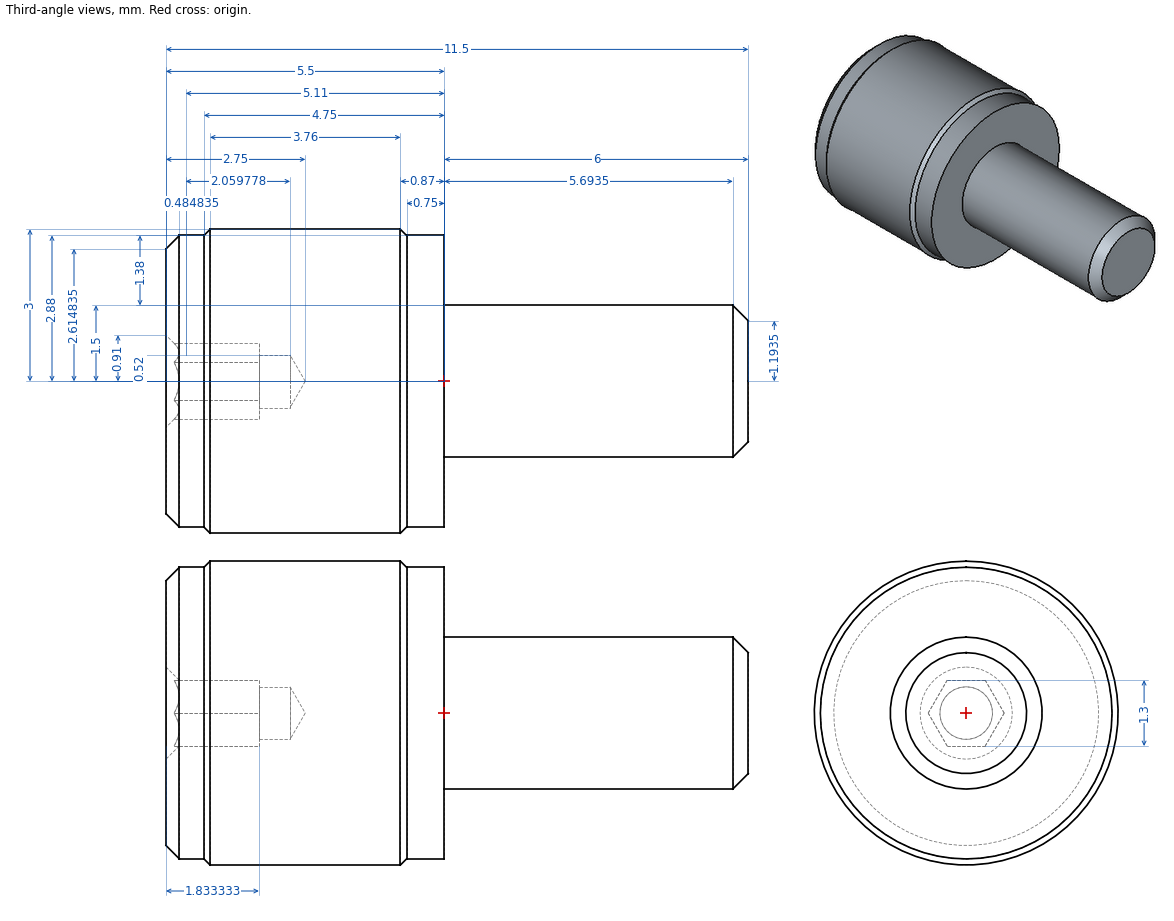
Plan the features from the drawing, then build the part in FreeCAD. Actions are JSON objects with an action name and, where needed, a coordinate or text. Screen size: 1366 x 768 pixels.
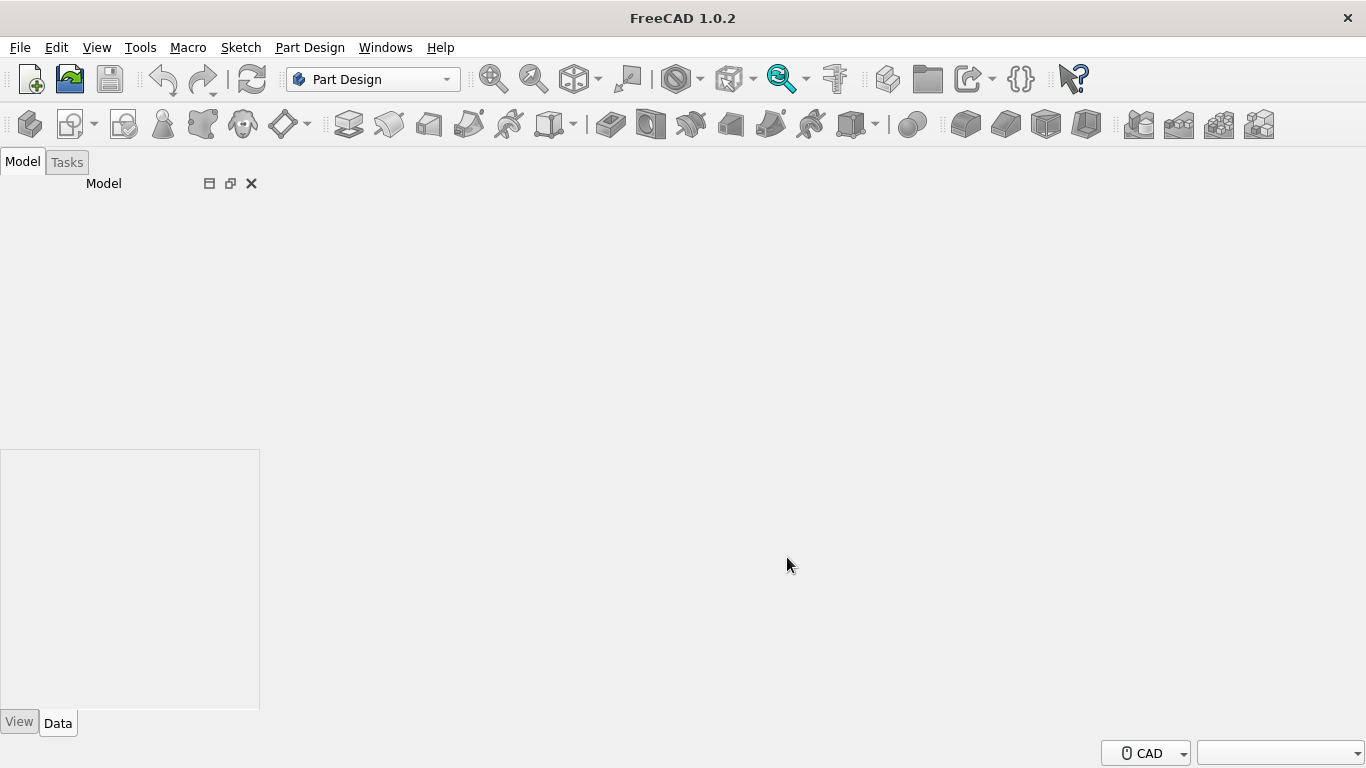
{"action": "left_click", "coordinate": [30, 80]}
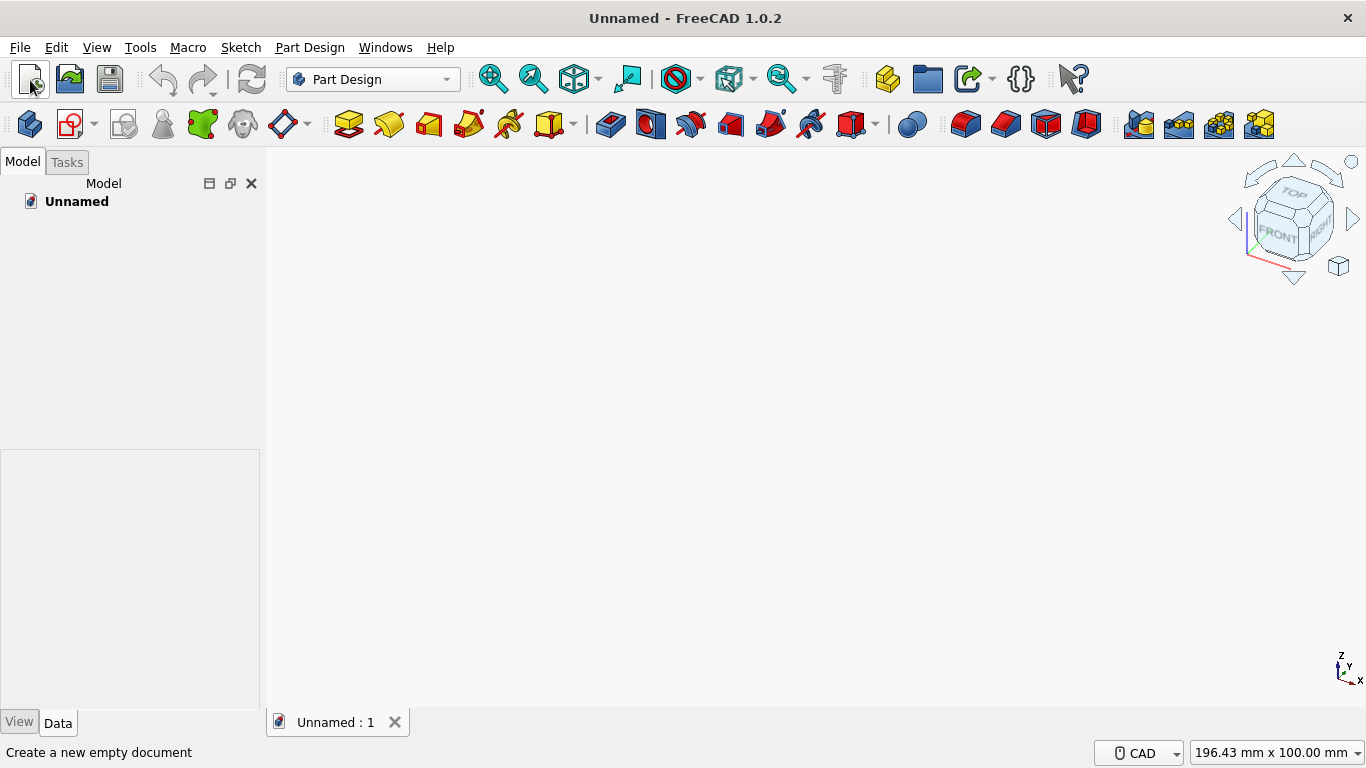
{"action": "left_click", "coordinate": [70, 124]}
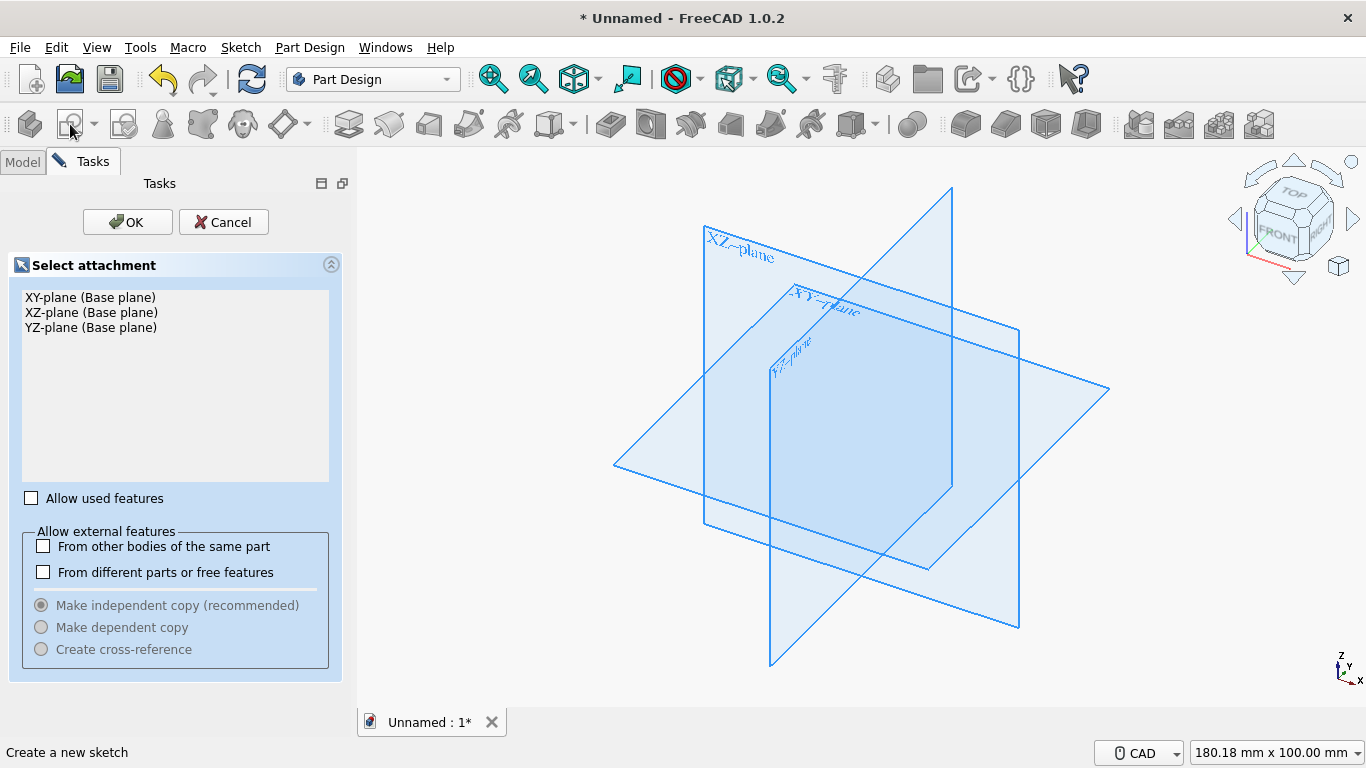
{"action": "left_click", "coordinate": [82, 298]}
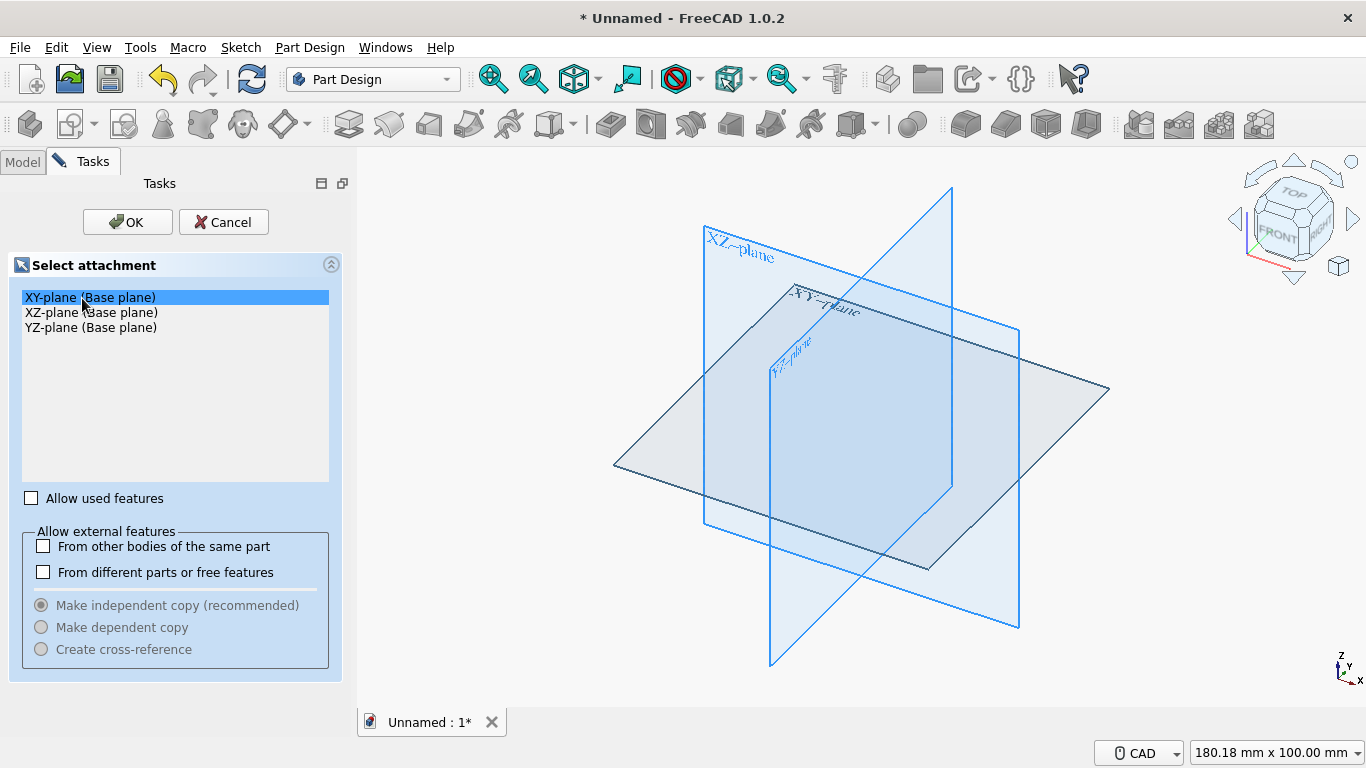
{"action": "left_click", "coordinate": [128, 222]}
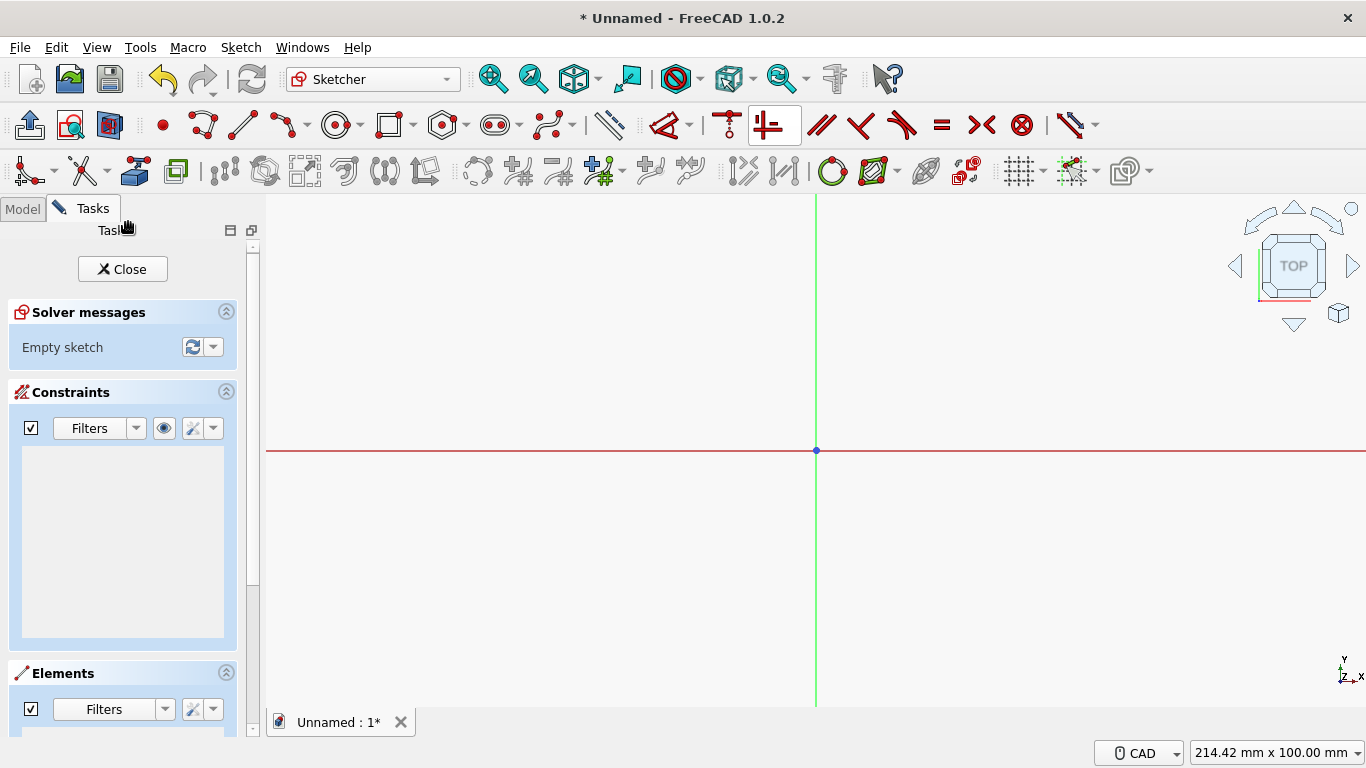
{"action": "scroll", "coordinate": [824, 442], "scroll_direction": "up", "scroll_amount": 12}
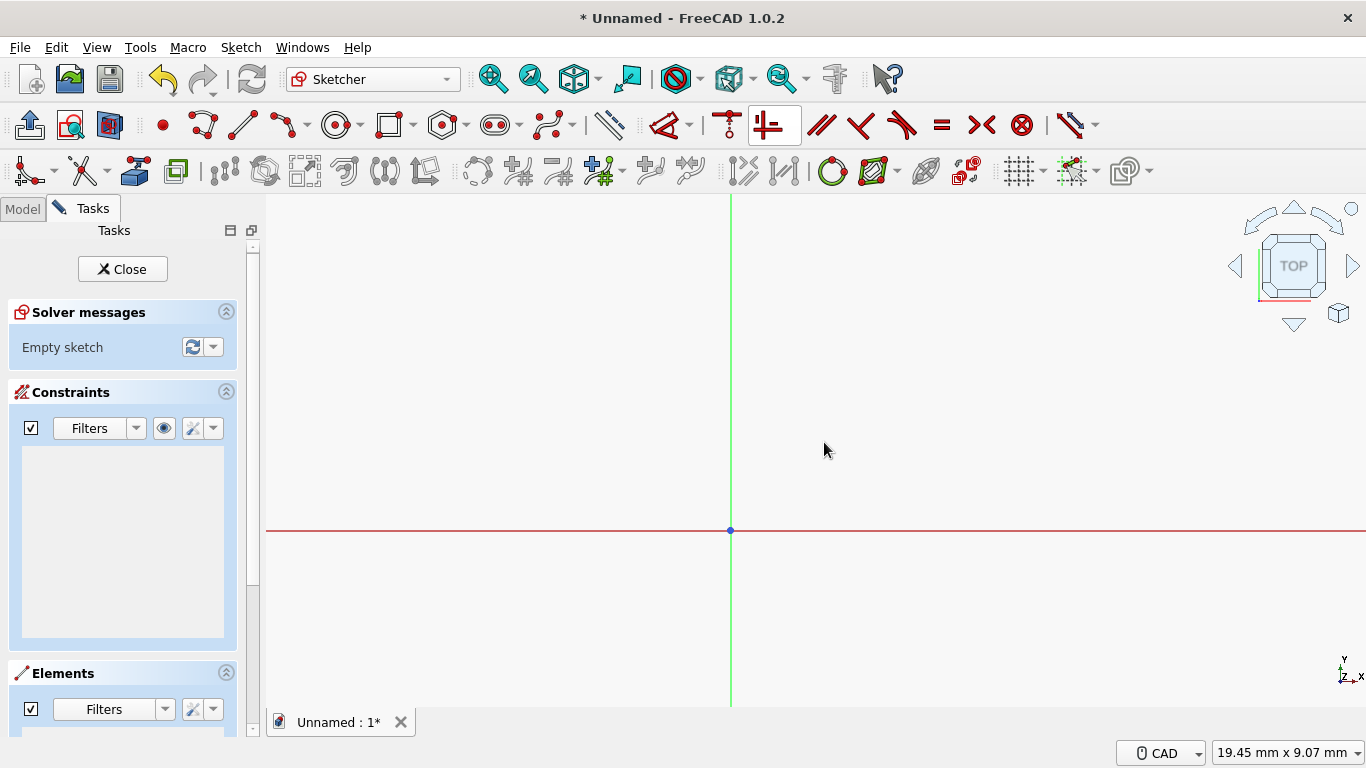
{"action": "left_click", "coordinate": [204, 126]}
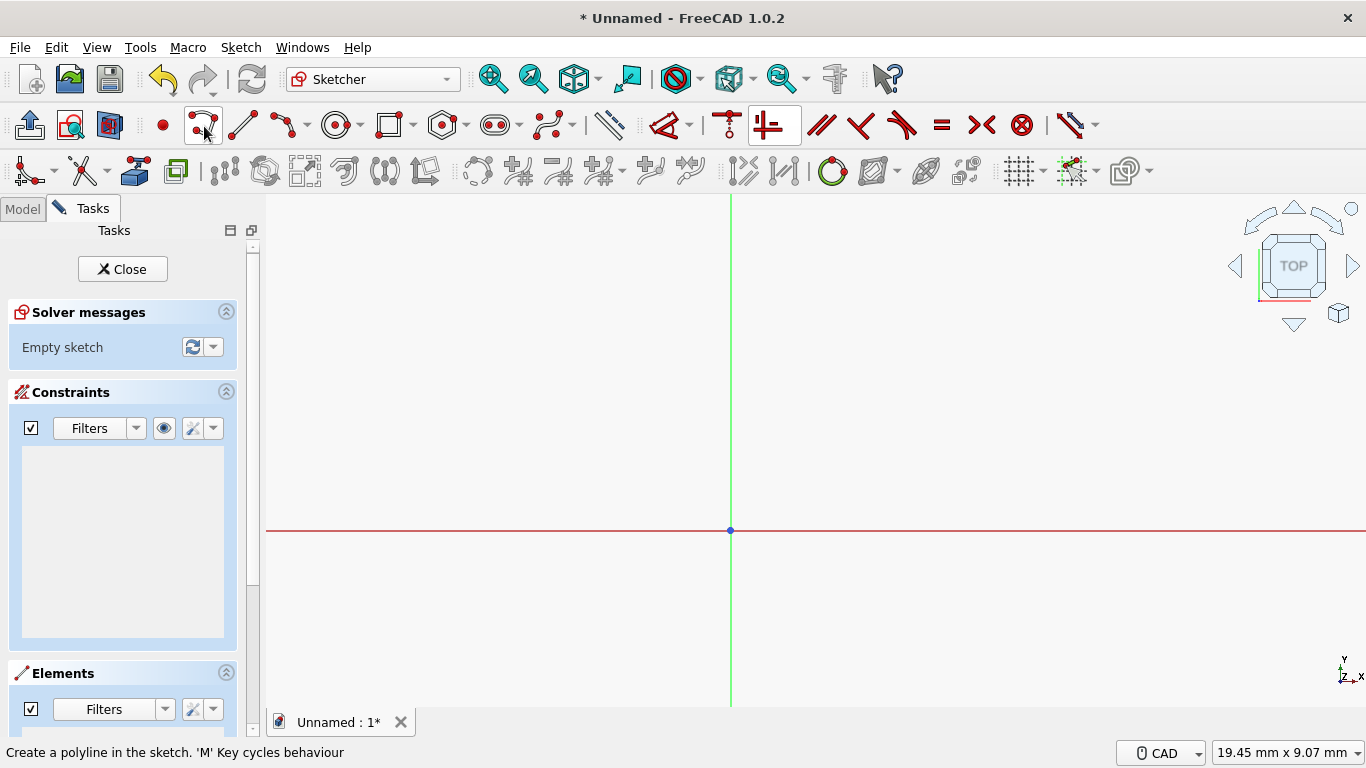
{"action": "left_click", "coordinate": [731, 446]}
{"action": "left_click", "coordinate": [740, 368]}
{"action": "left_click", "coordinate": [688, 368]}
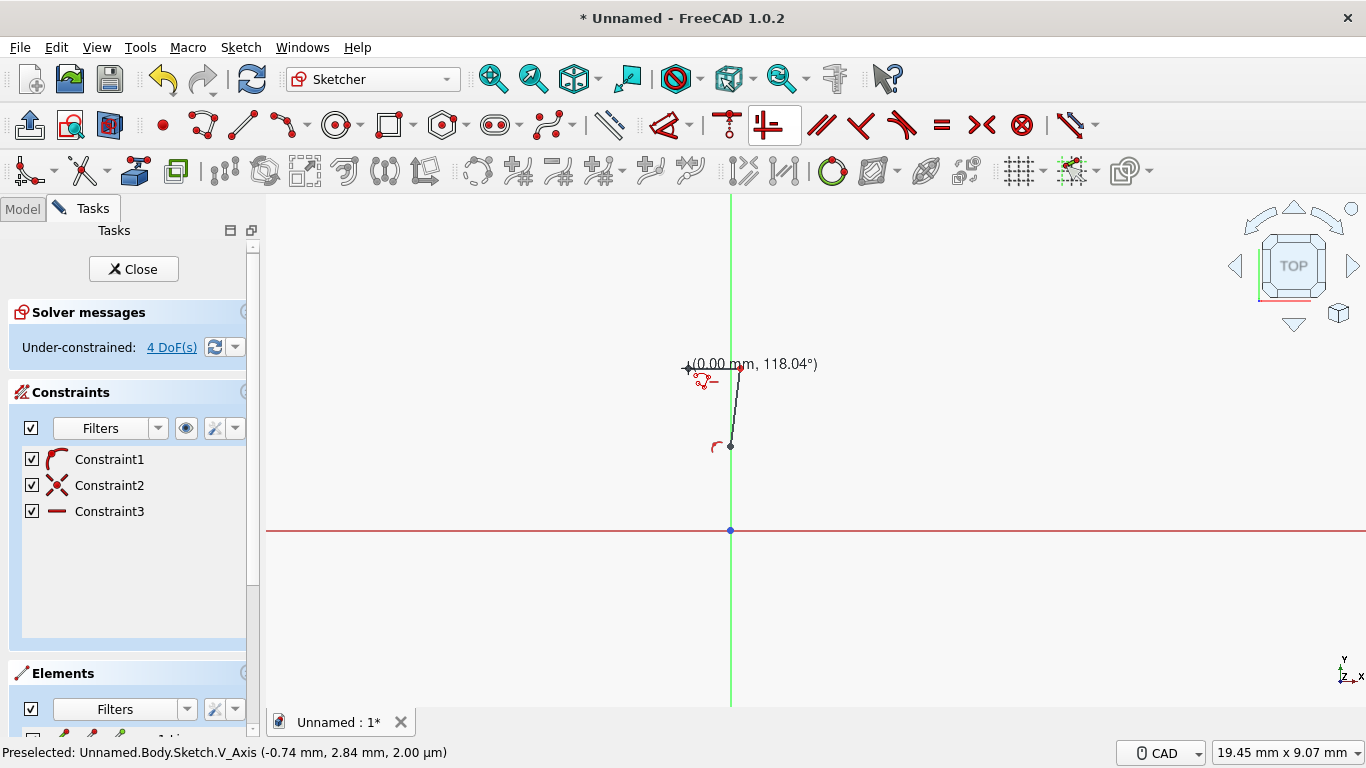
{"action": "scroll", "coordinate": [682, 361], "scroll_direction": "up", "scroll_amount": 3}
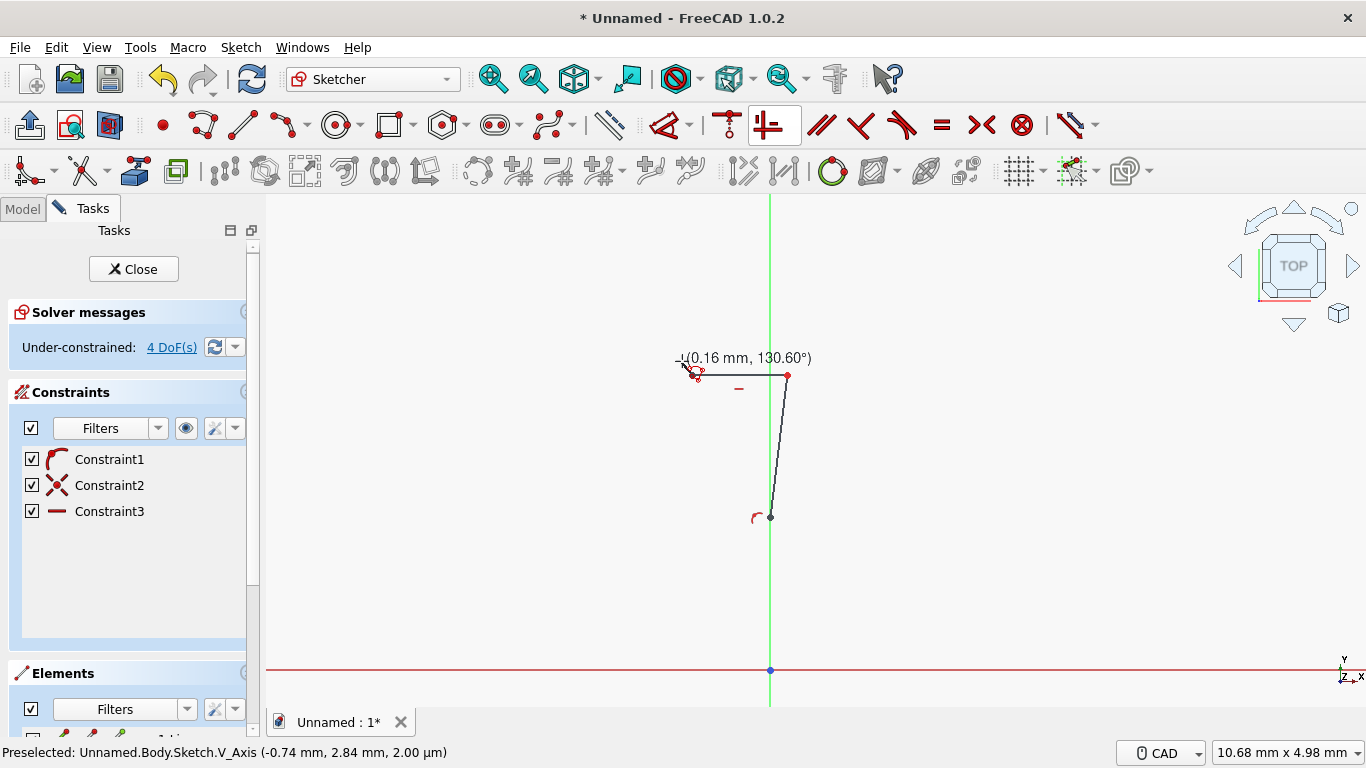
{"action": "left_click", "coordinate": [681, 361]}